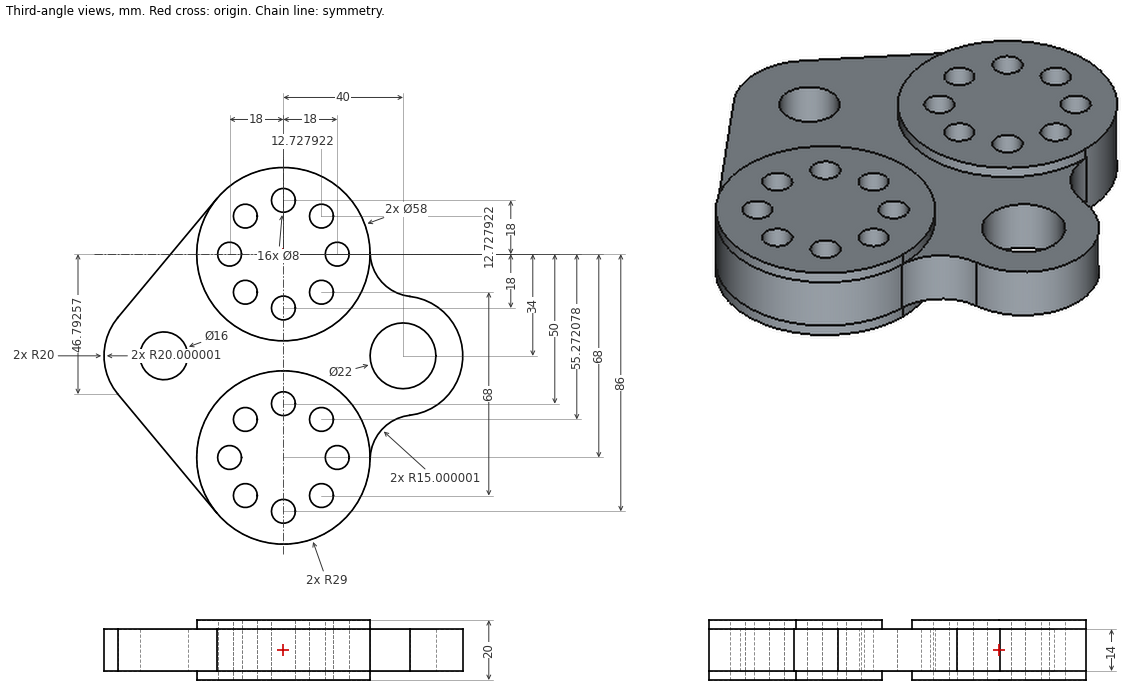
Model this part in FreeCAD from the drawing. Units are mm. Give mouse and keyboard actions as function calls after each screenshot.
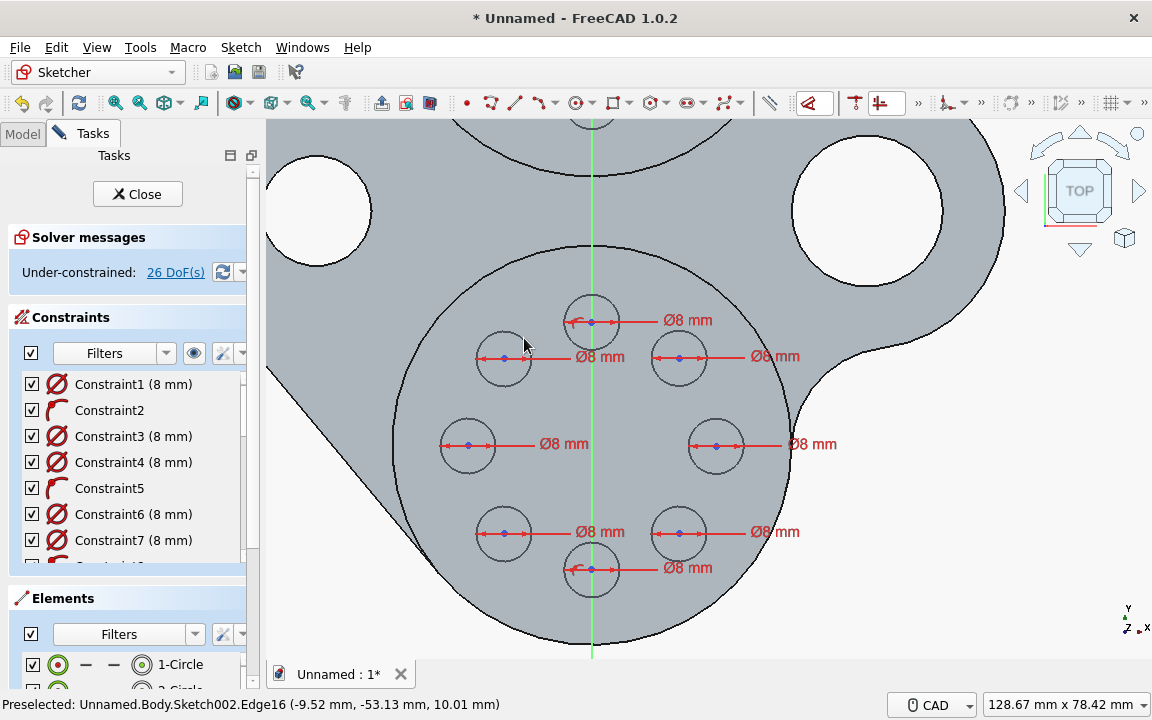
scroll(680, 534, down, 4)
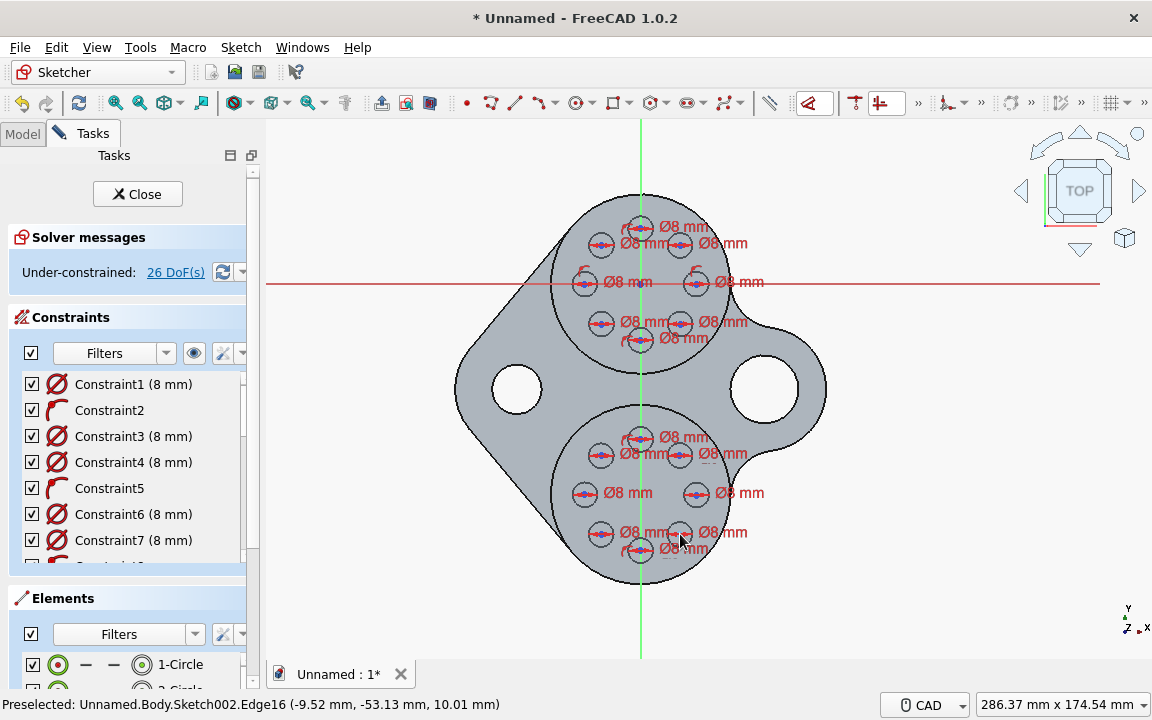
click(680, 245)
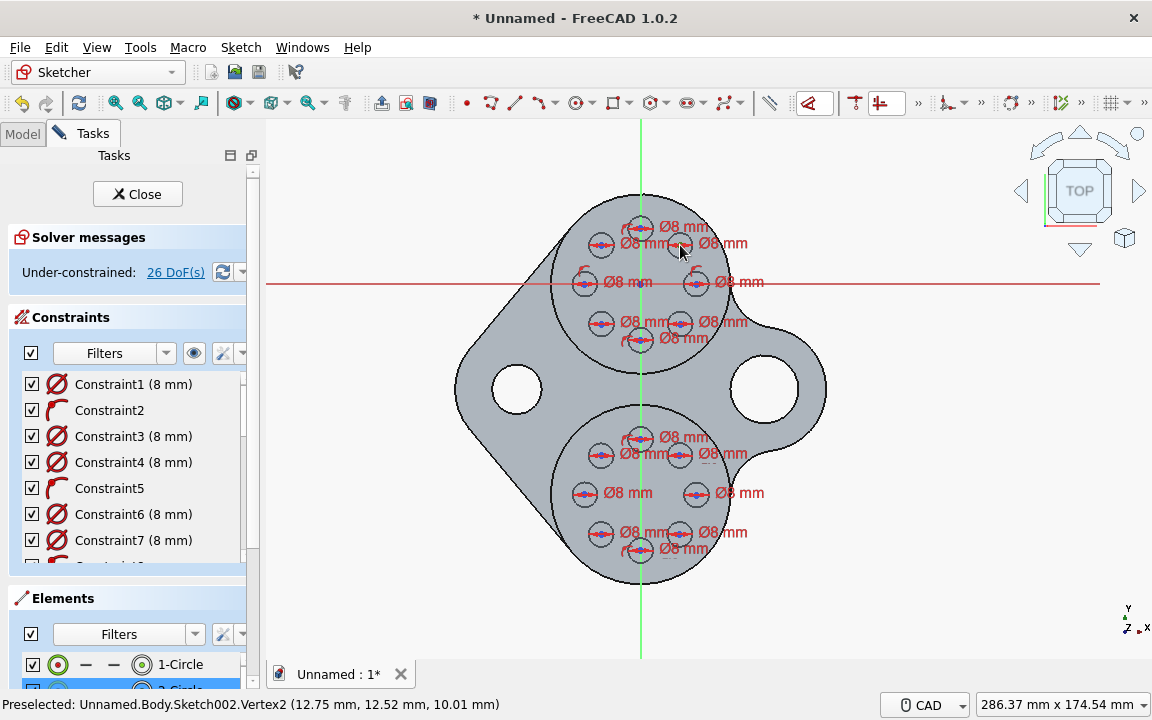
click(680, 324)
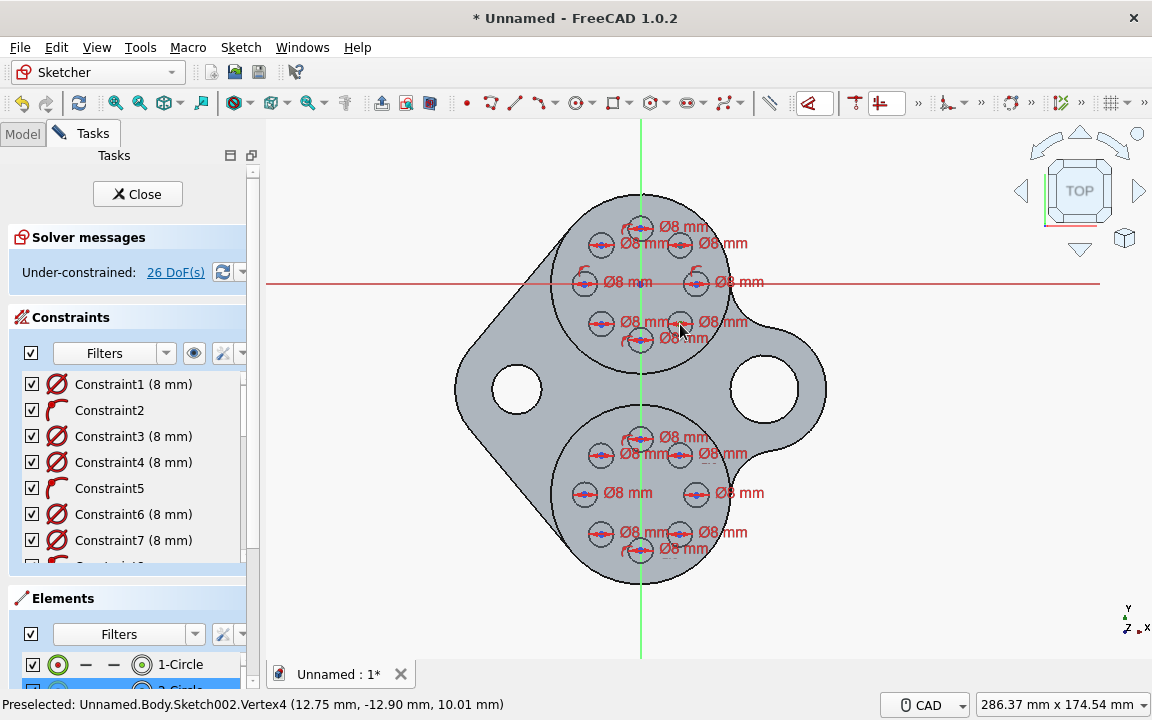
click(344, 284)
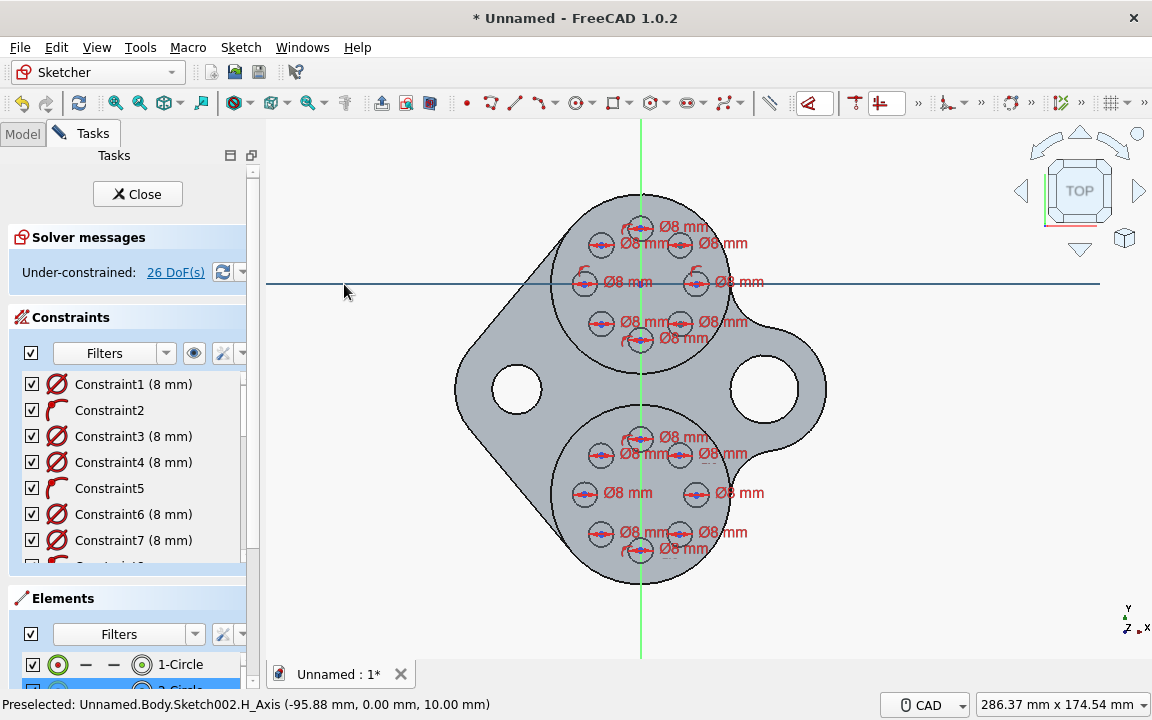
key(s)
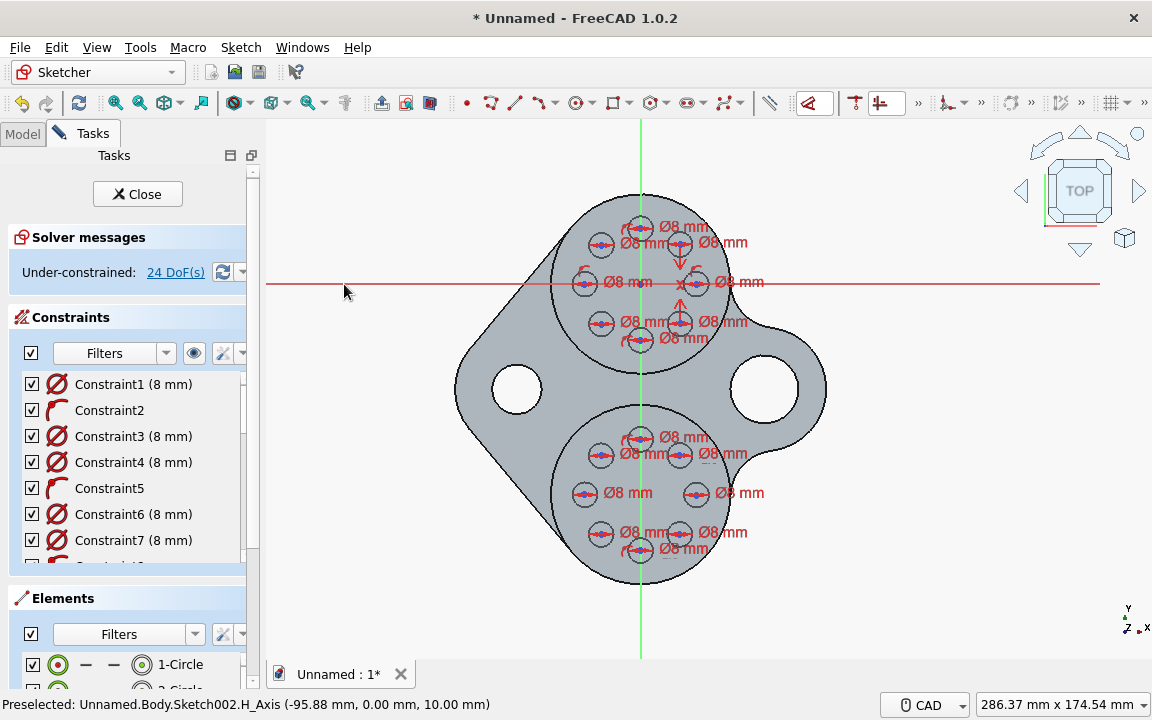
click(680, 324)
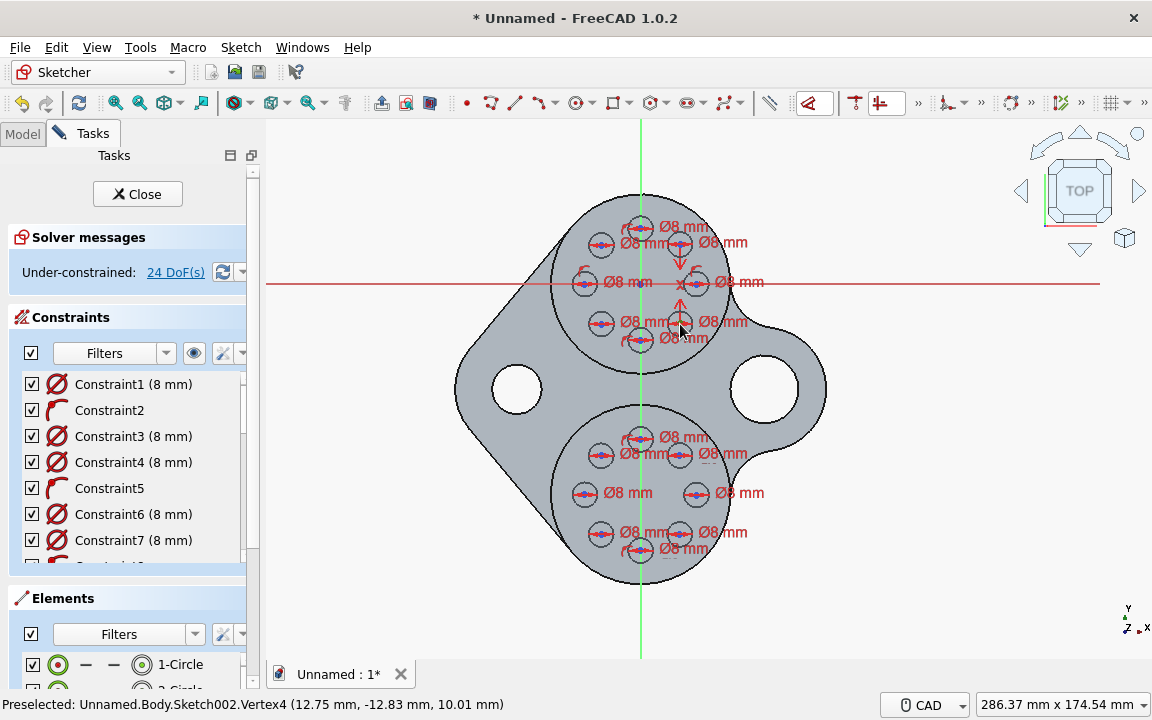
click(601, 324)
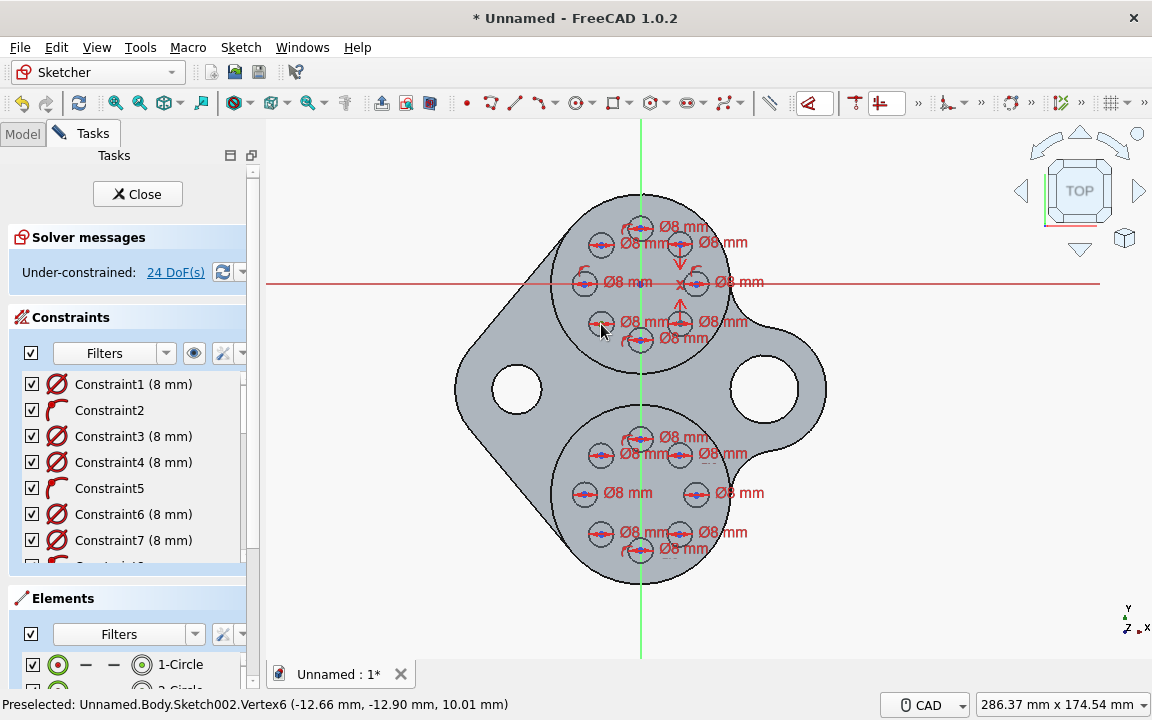
click(641, 596)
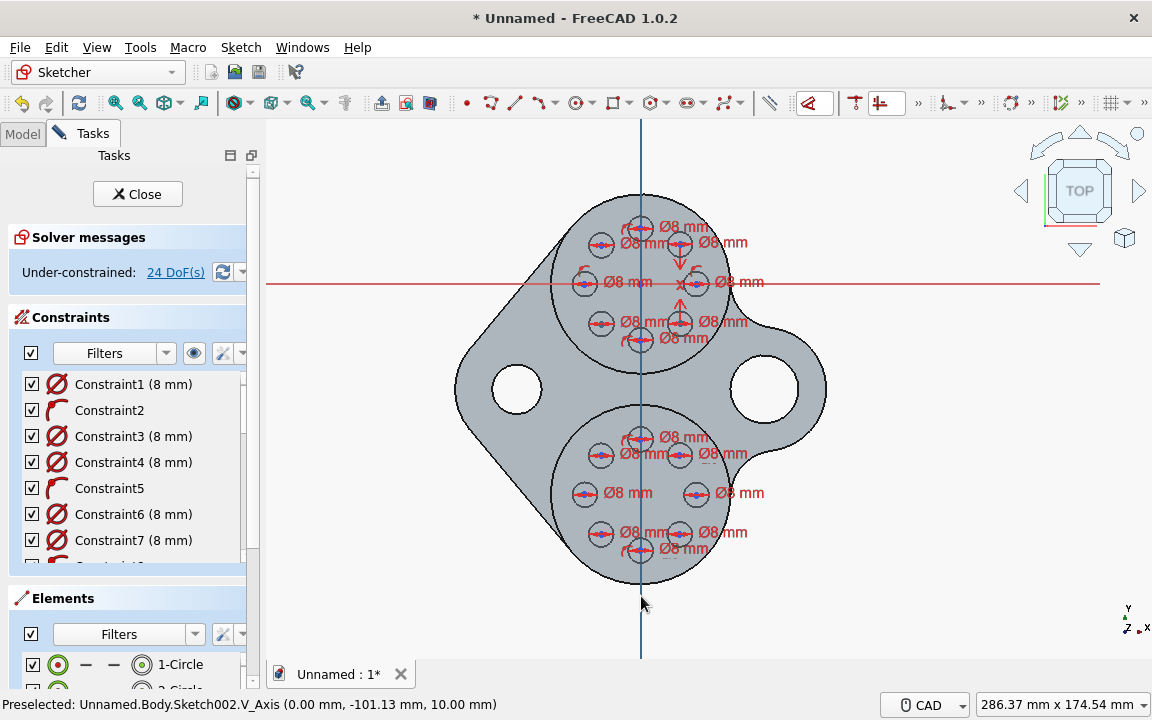
key(s)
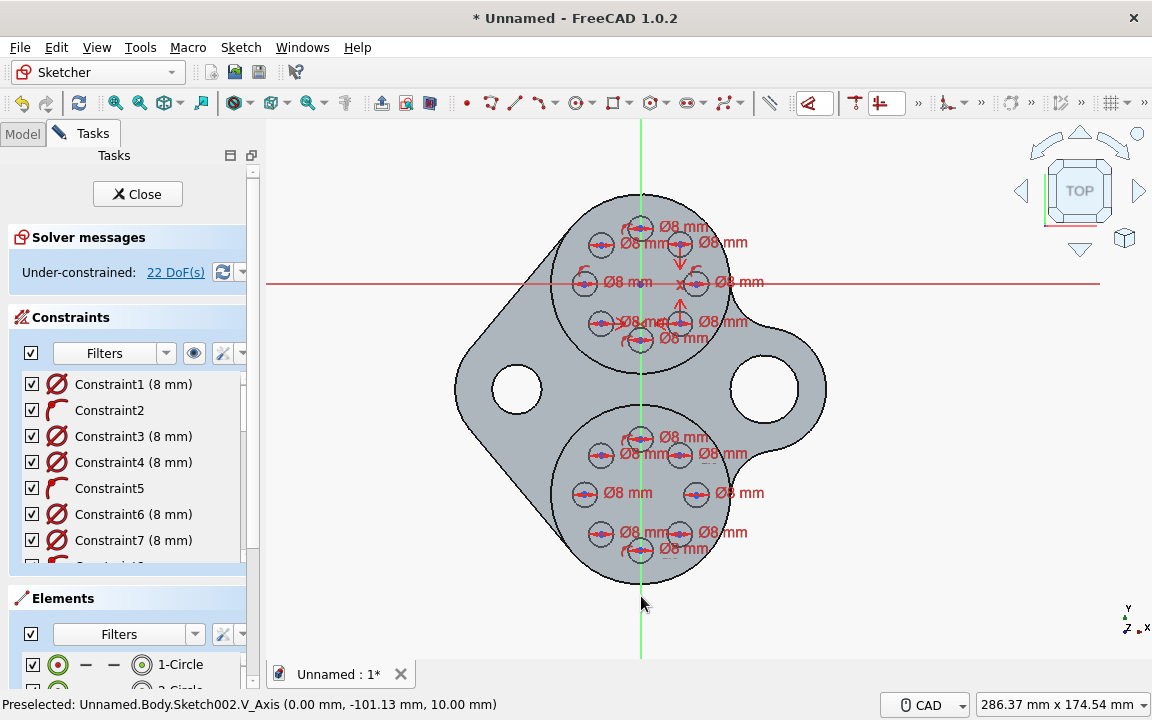
click(680, 244)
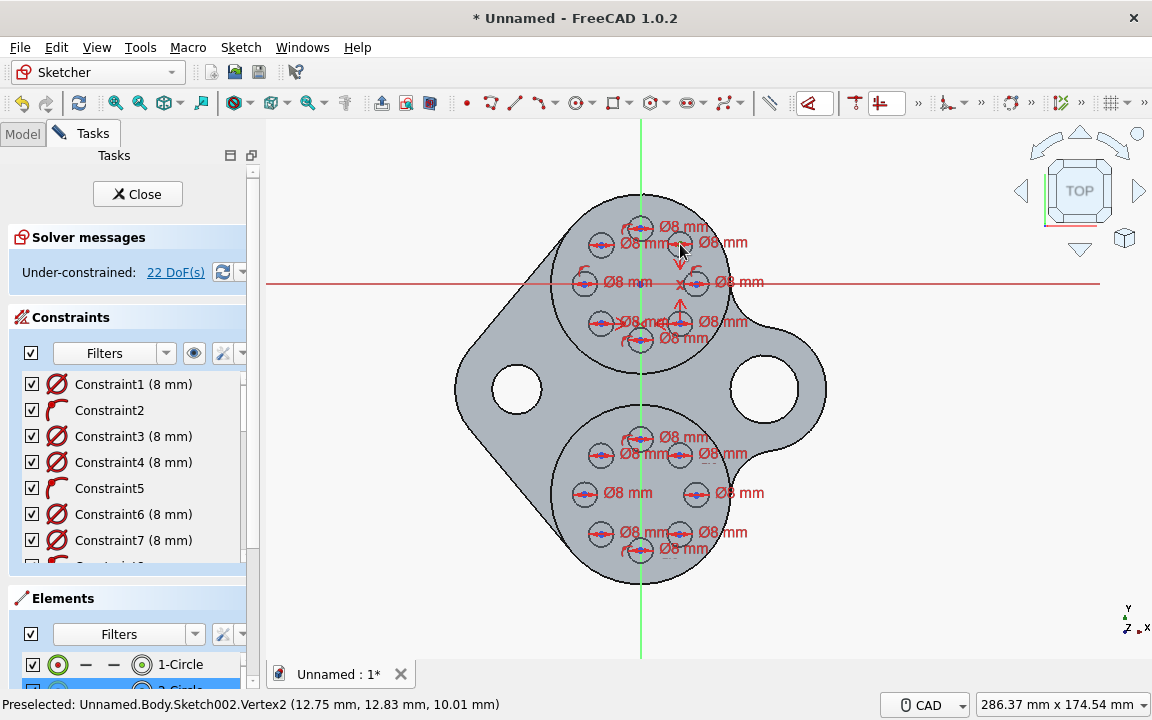
click(601, 245)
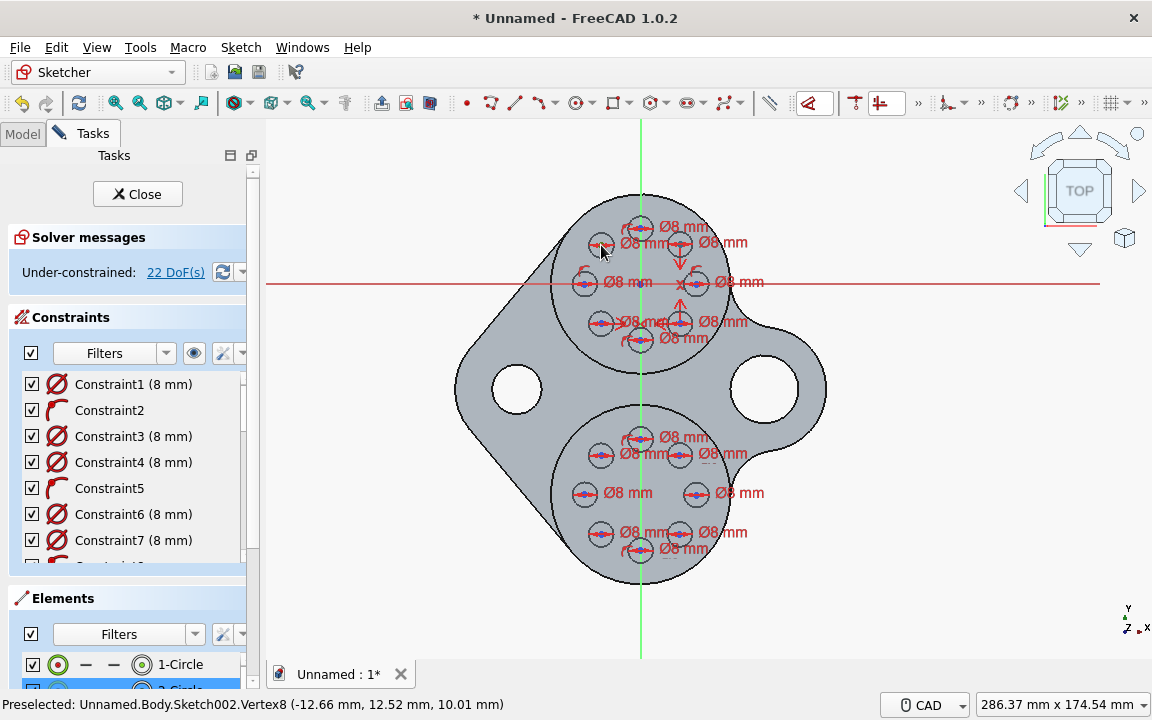
click(641, 596)